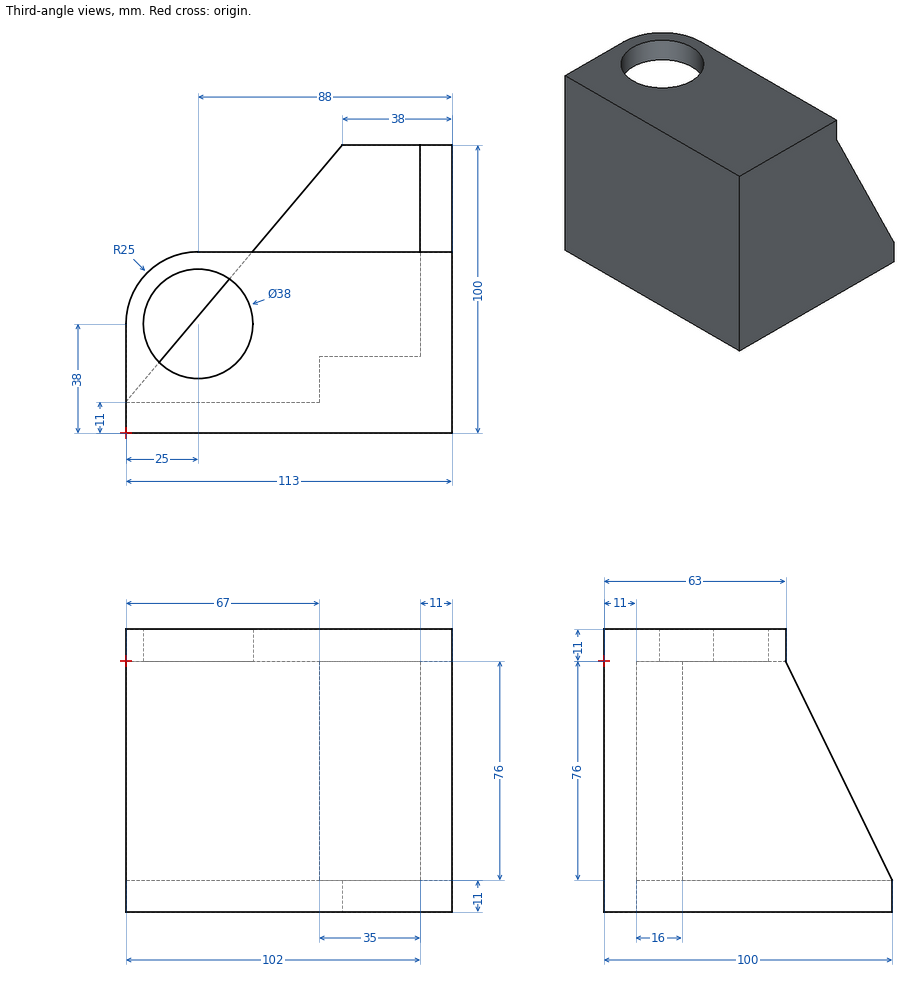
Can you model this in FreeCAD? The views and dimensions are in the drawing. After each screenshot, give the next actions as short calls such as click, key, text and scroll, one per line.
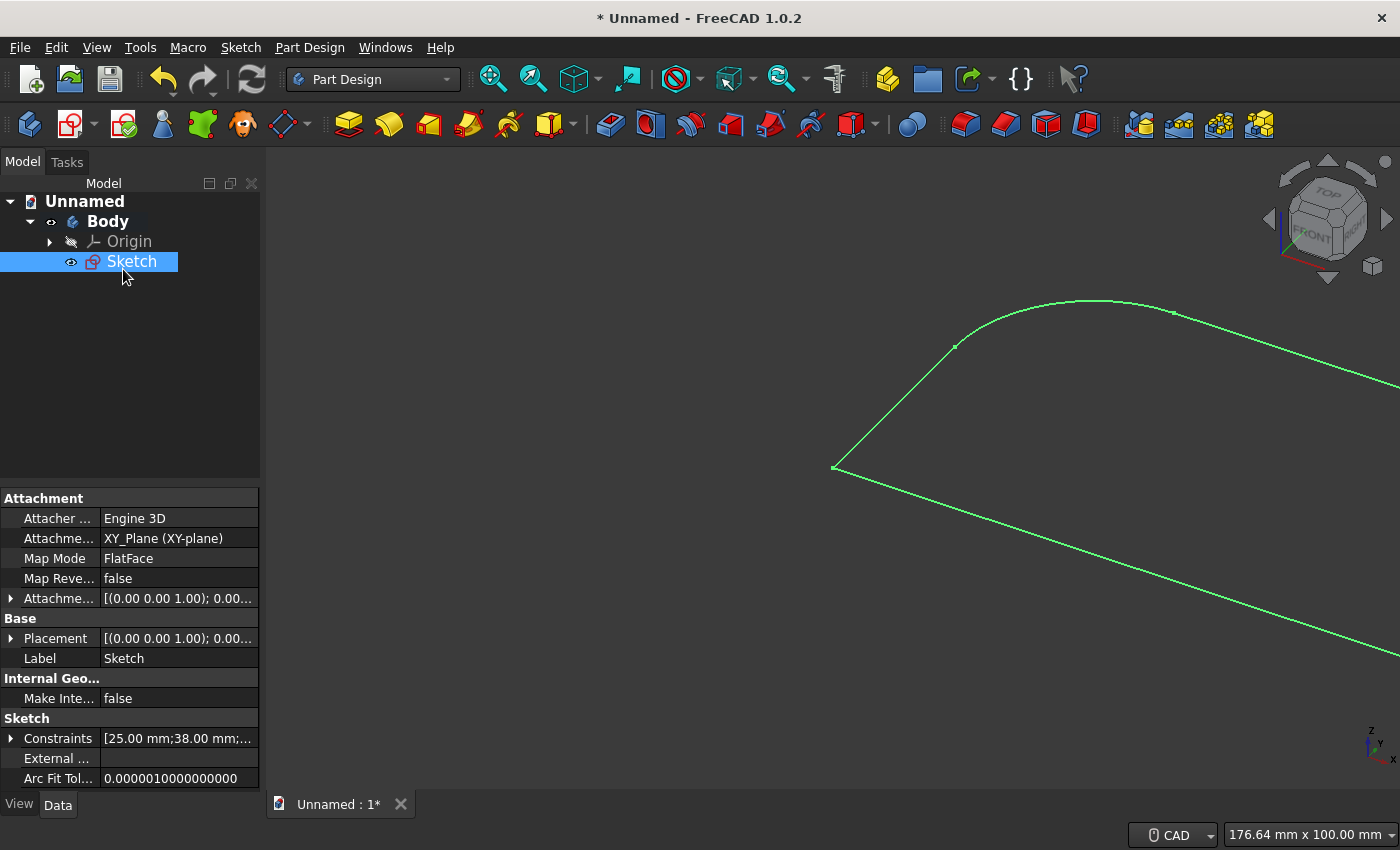
click(350, 124)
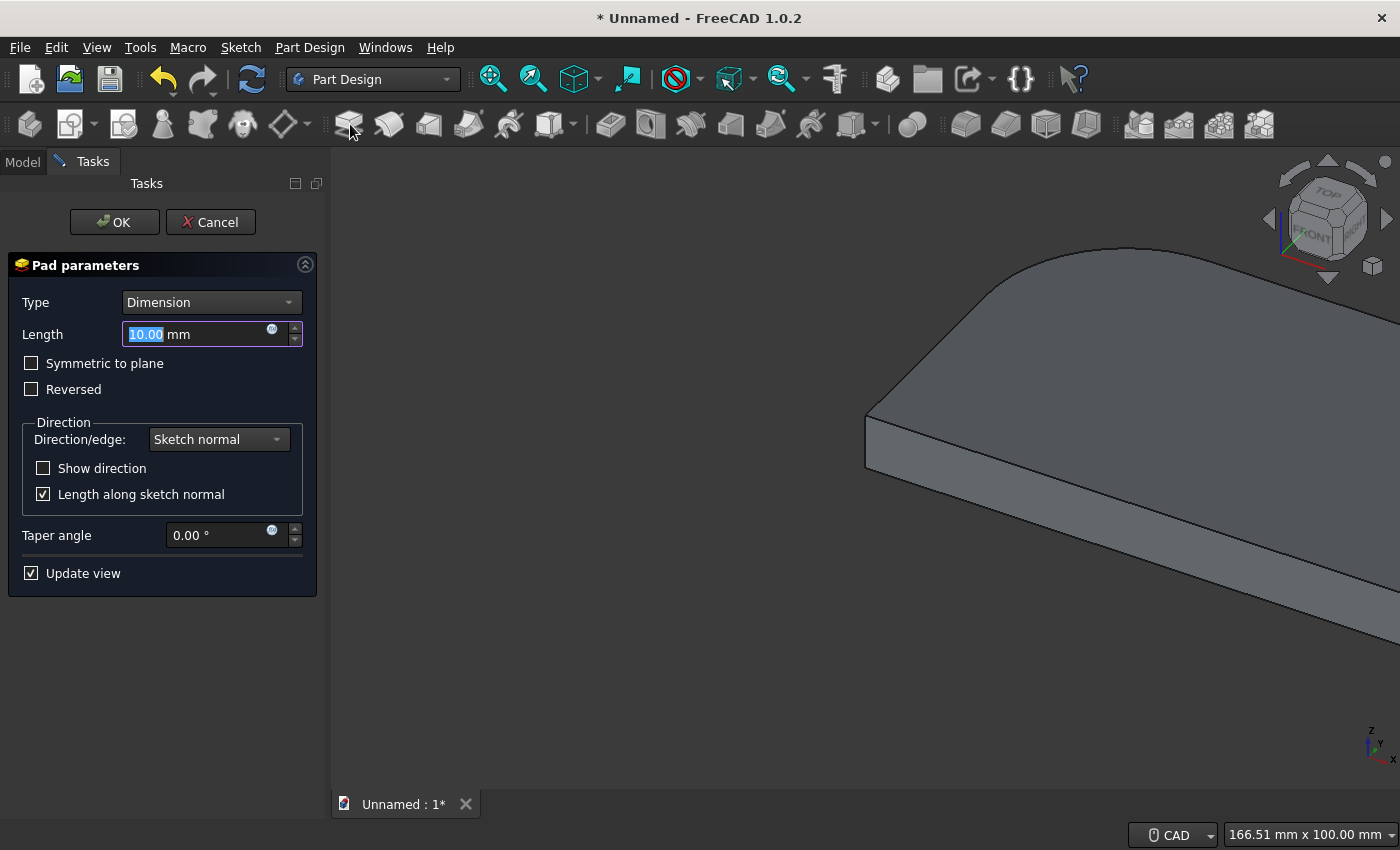
text(11)
key(Tab)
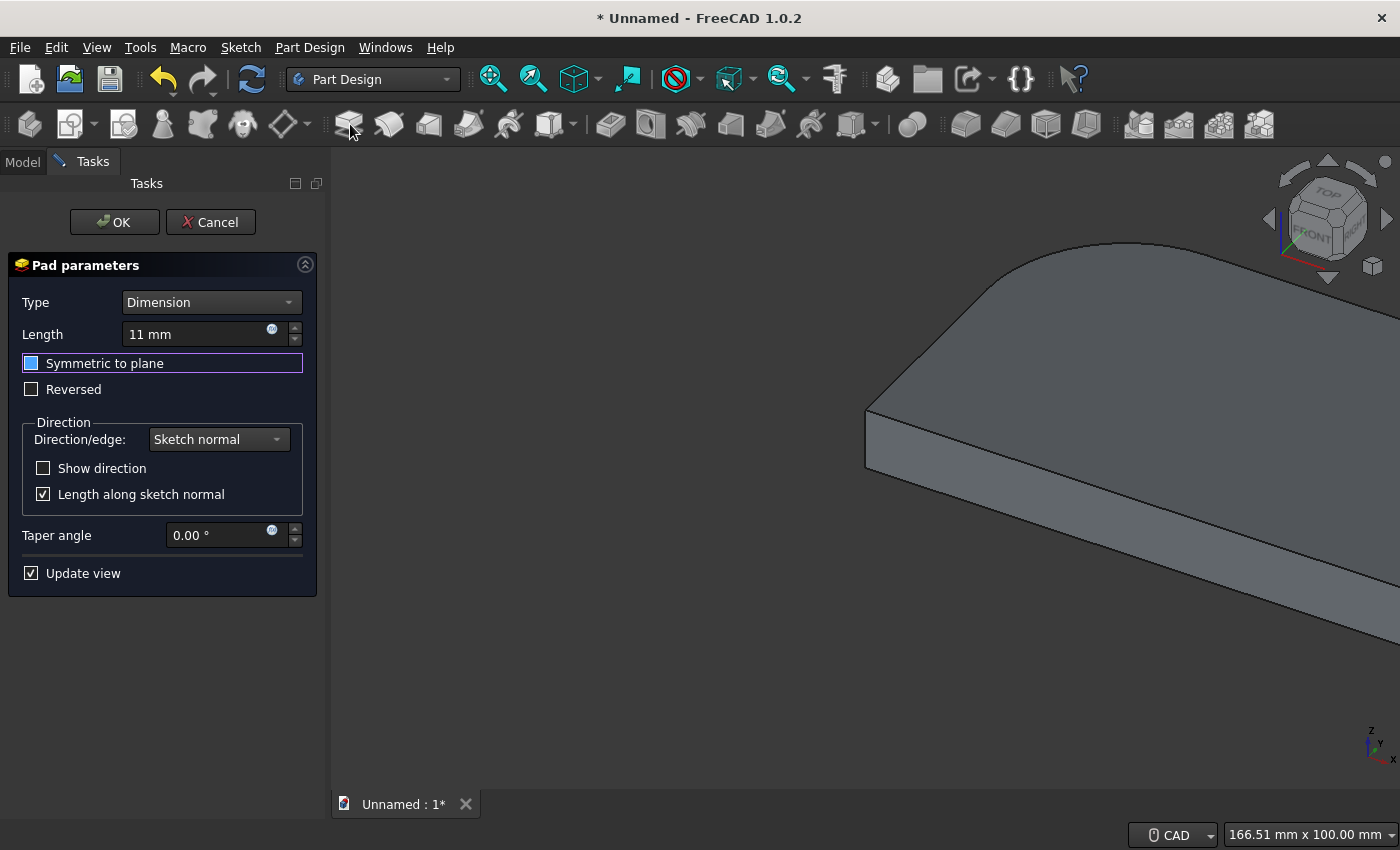
click(115, 222)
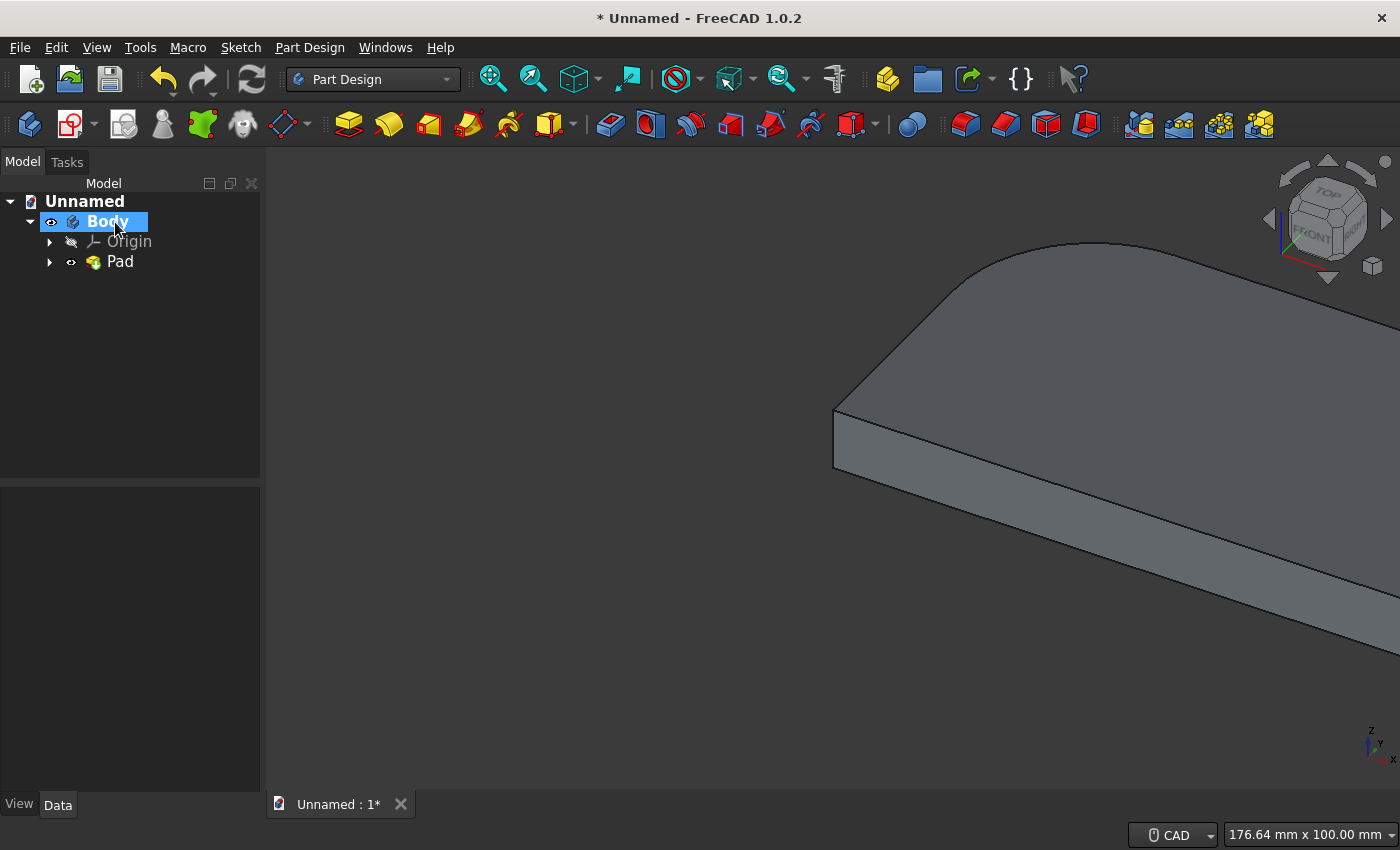
key(v)
key(f)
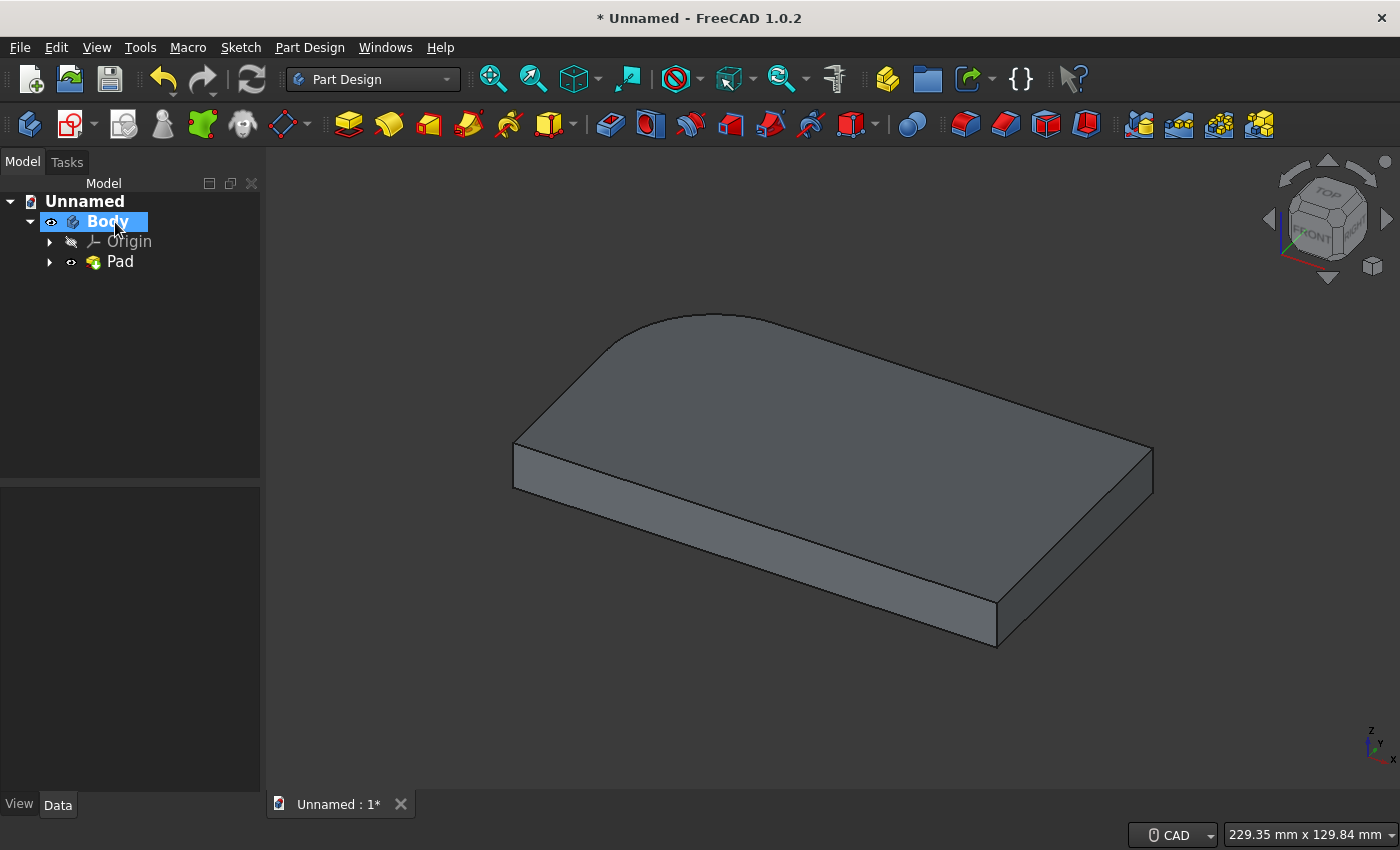
click(1119, 503)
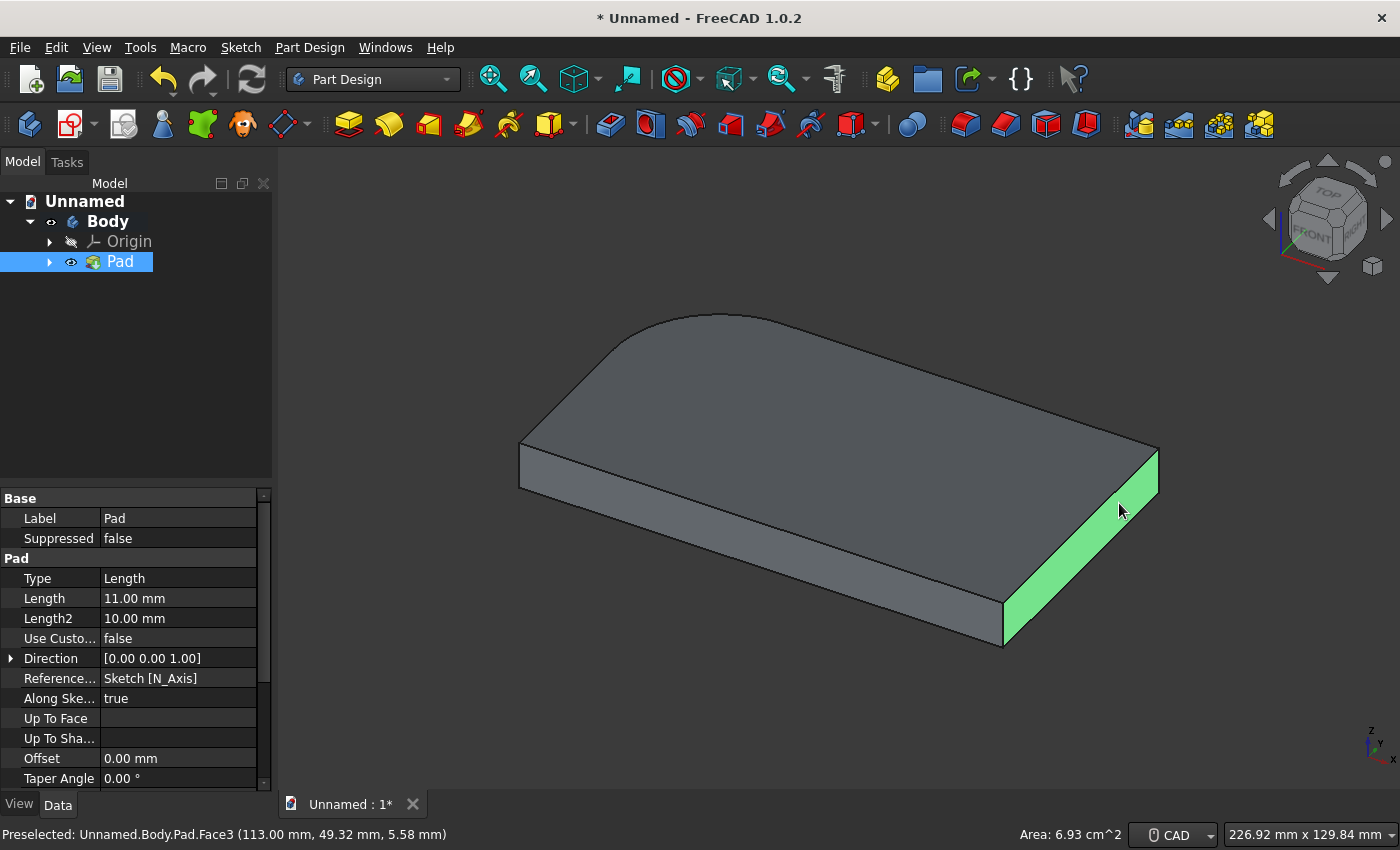
click(70, 124)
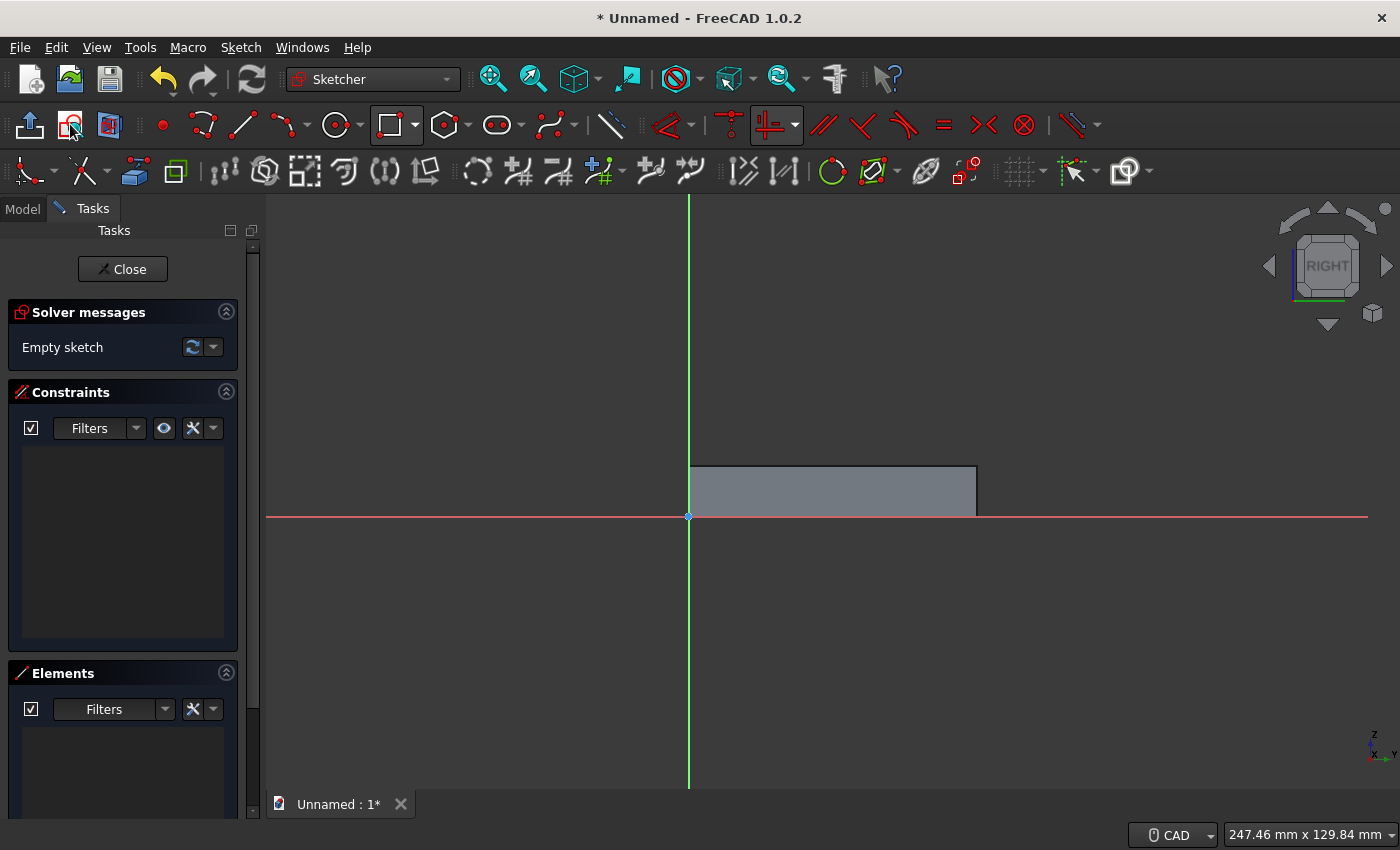
scroll(453, 222, down, 2)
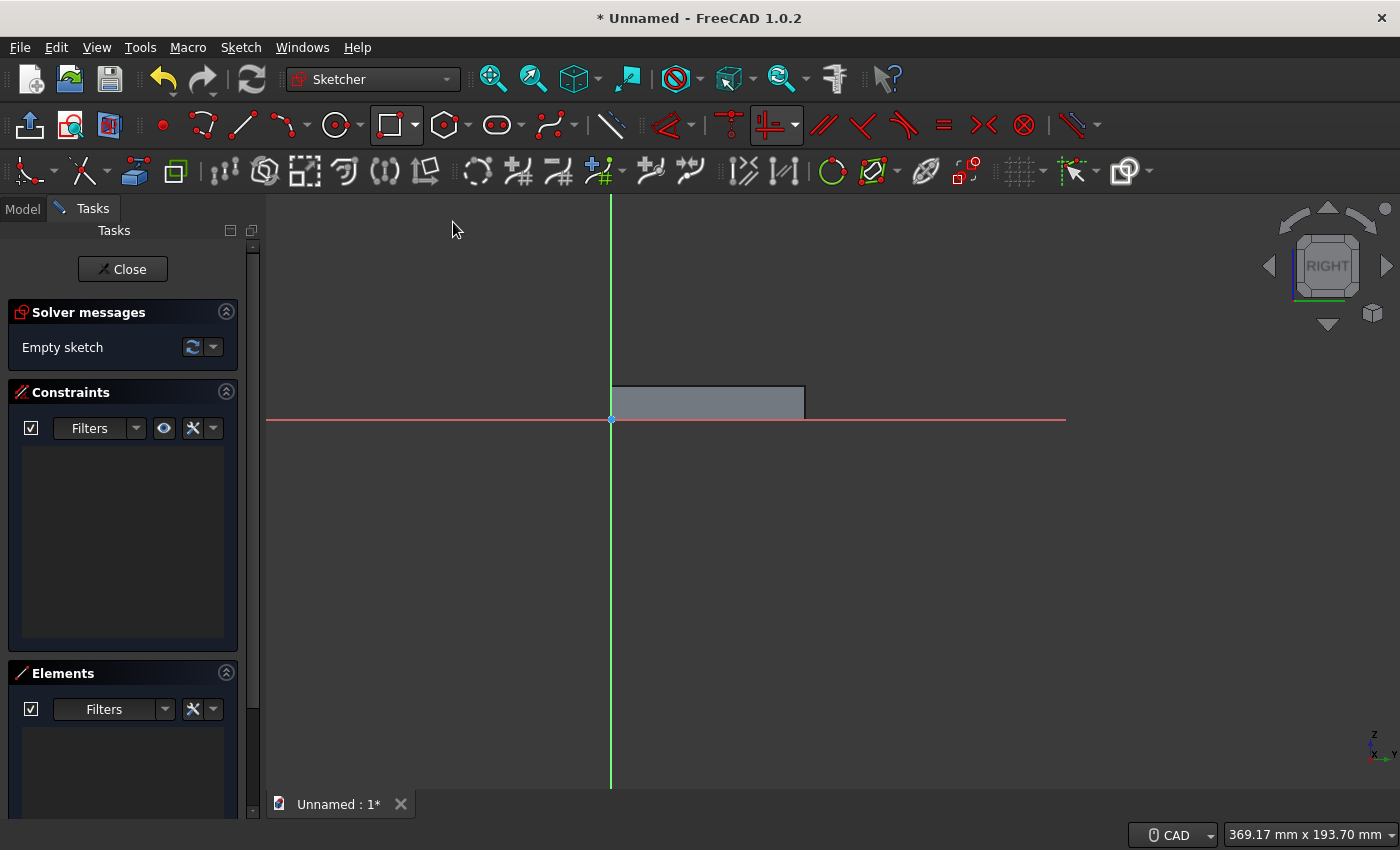
scroll(765, 627, up, 2)